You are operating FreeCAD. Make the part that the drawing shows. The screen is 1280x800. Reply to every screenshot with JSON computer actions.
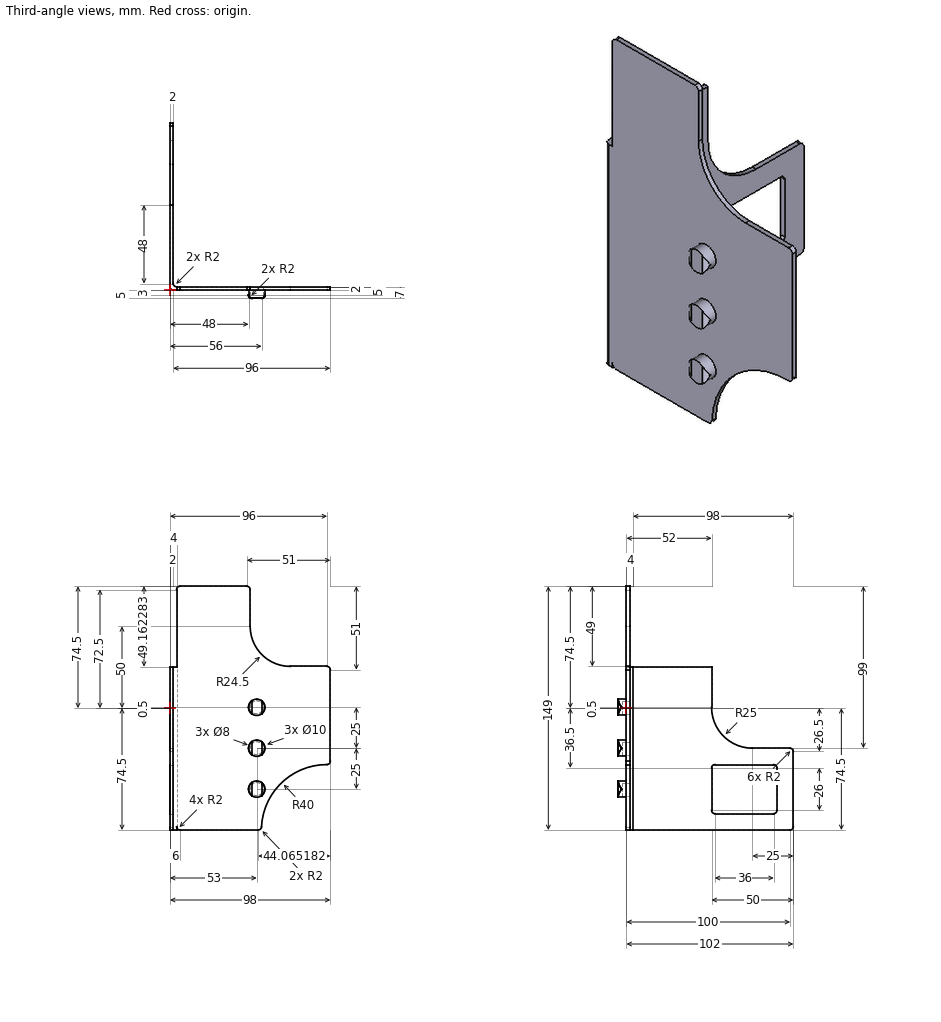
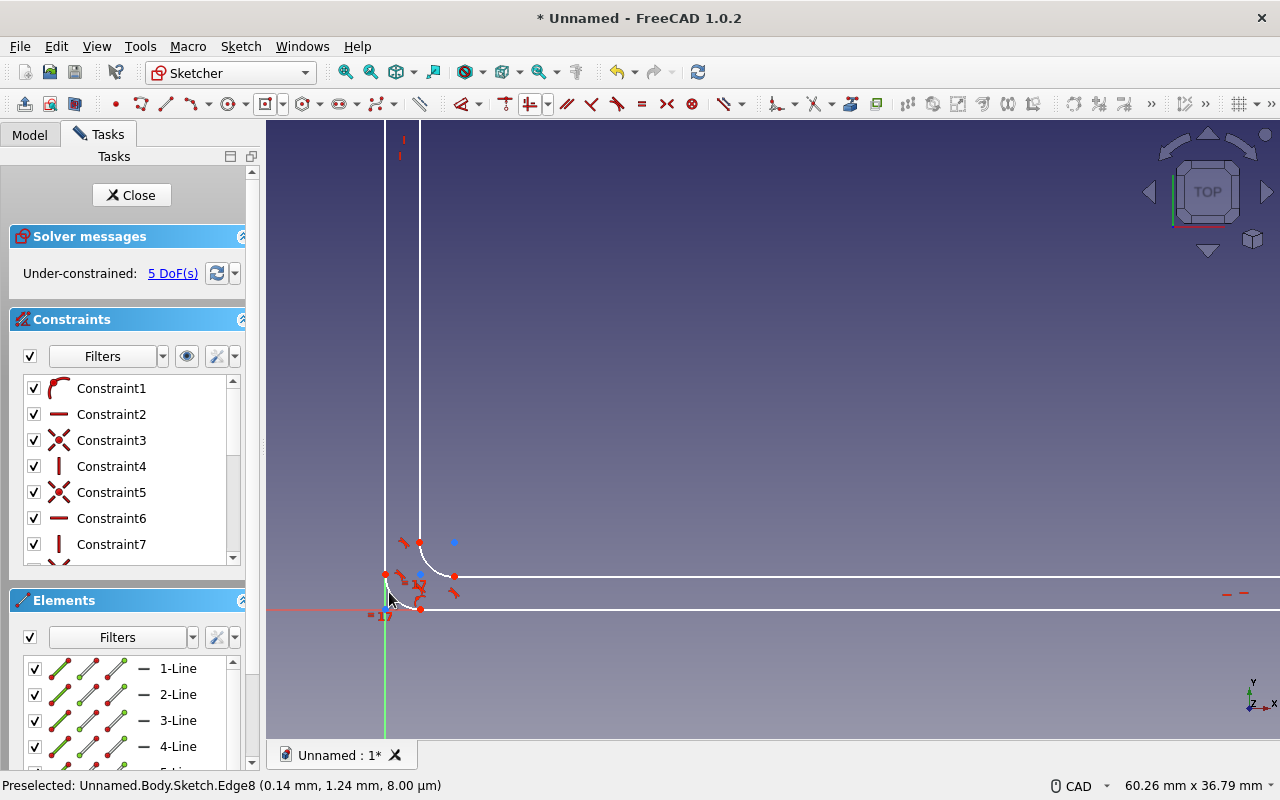
{"action": "left_click", "coordinate": [424, 558]}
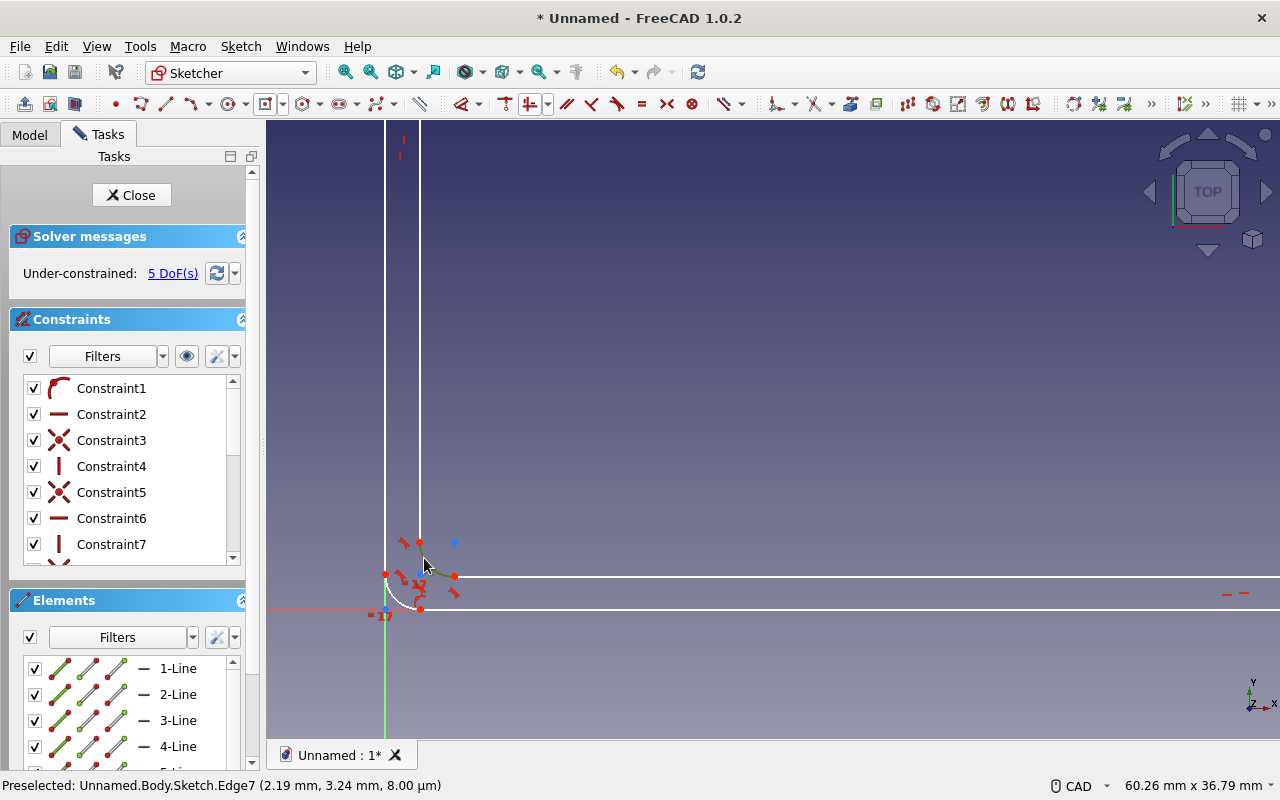
{"action": "key", "text": "k r"}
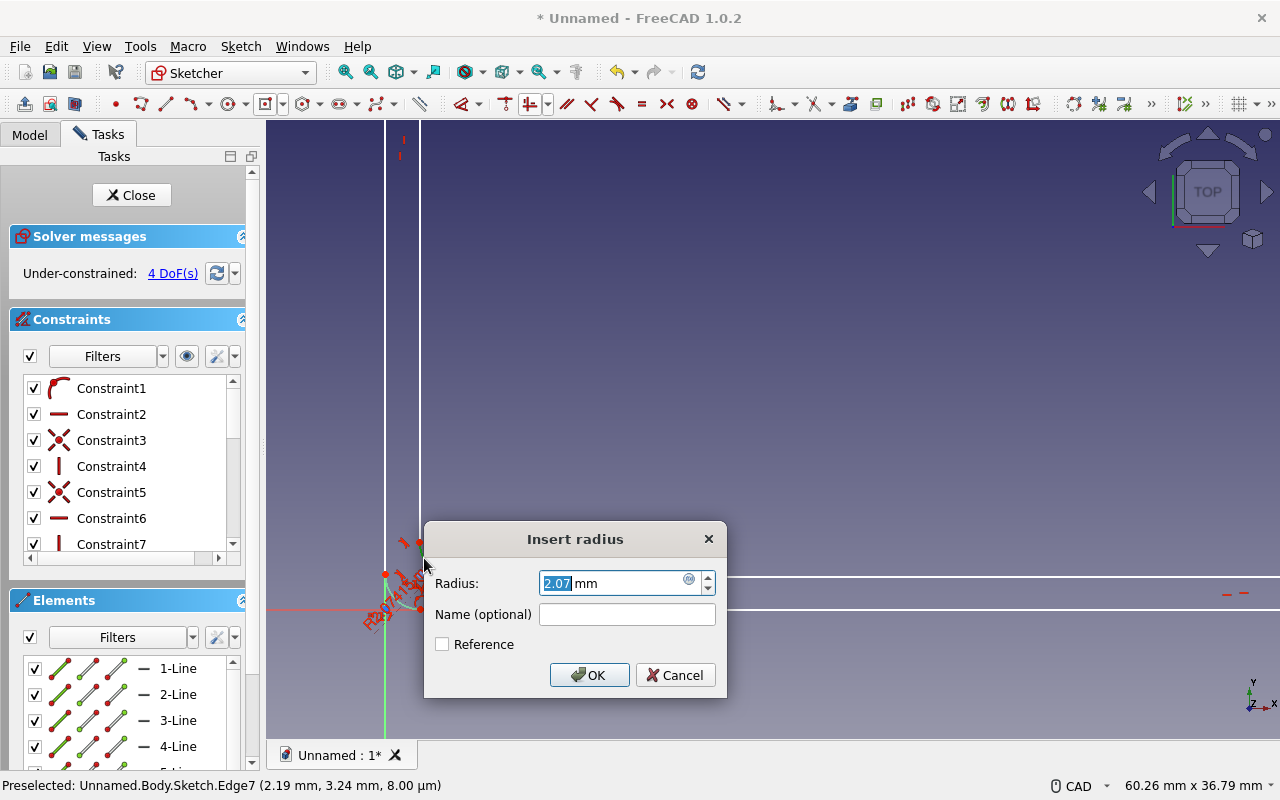
{"action": "type", "text": "2"}
{"action": "key", "text": "Return"}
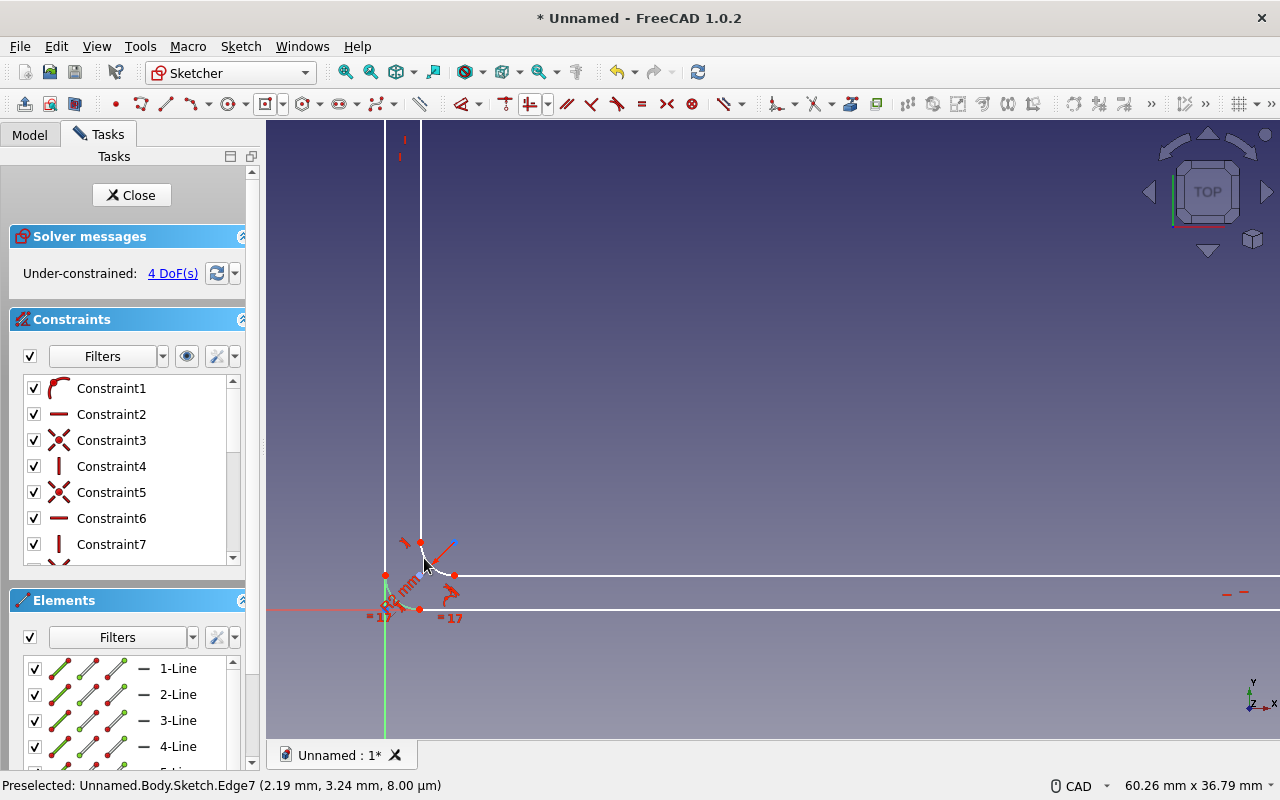
{"action": "scroll", "coordinate": [410, 579], "scroll_direction": "down", "scroll_amount": 5}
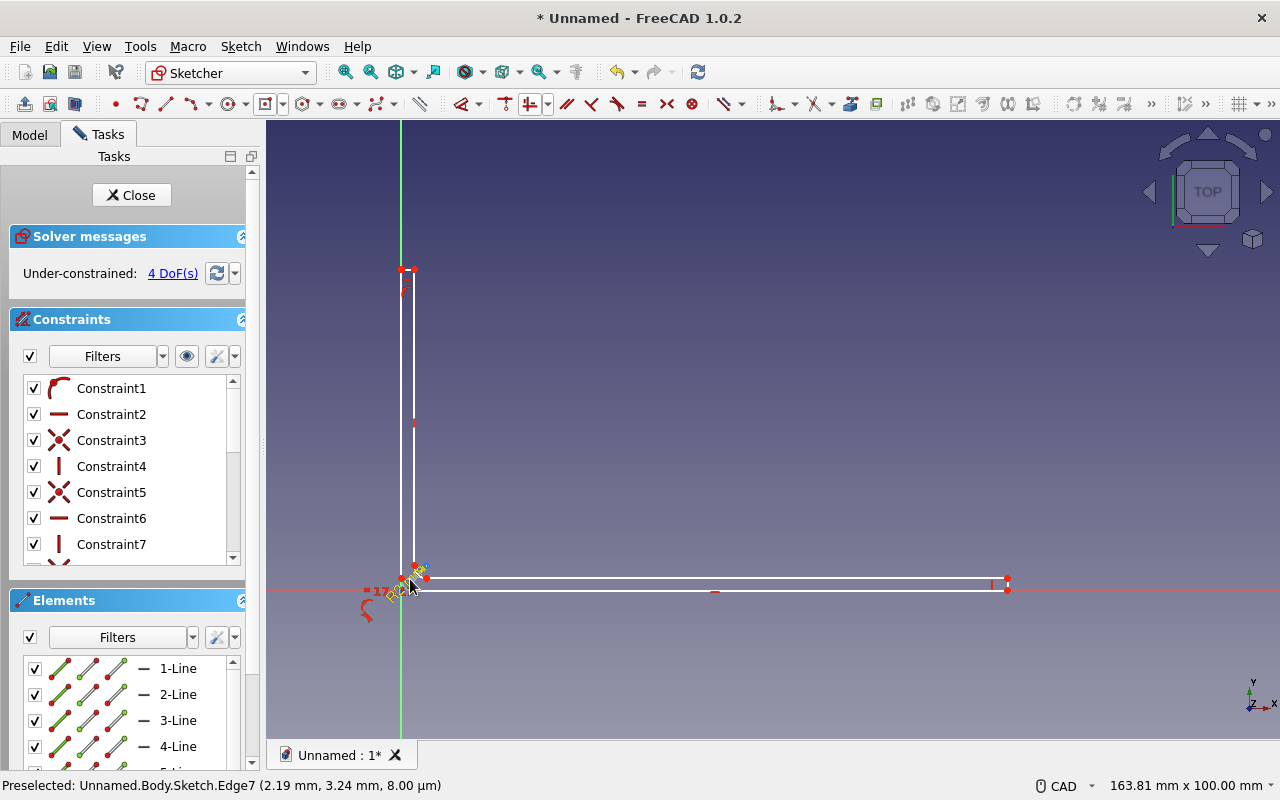
{"action": "scroll", "coordinate": [1008, 587], "scroll_direction": "up", "scroll_amount": 7}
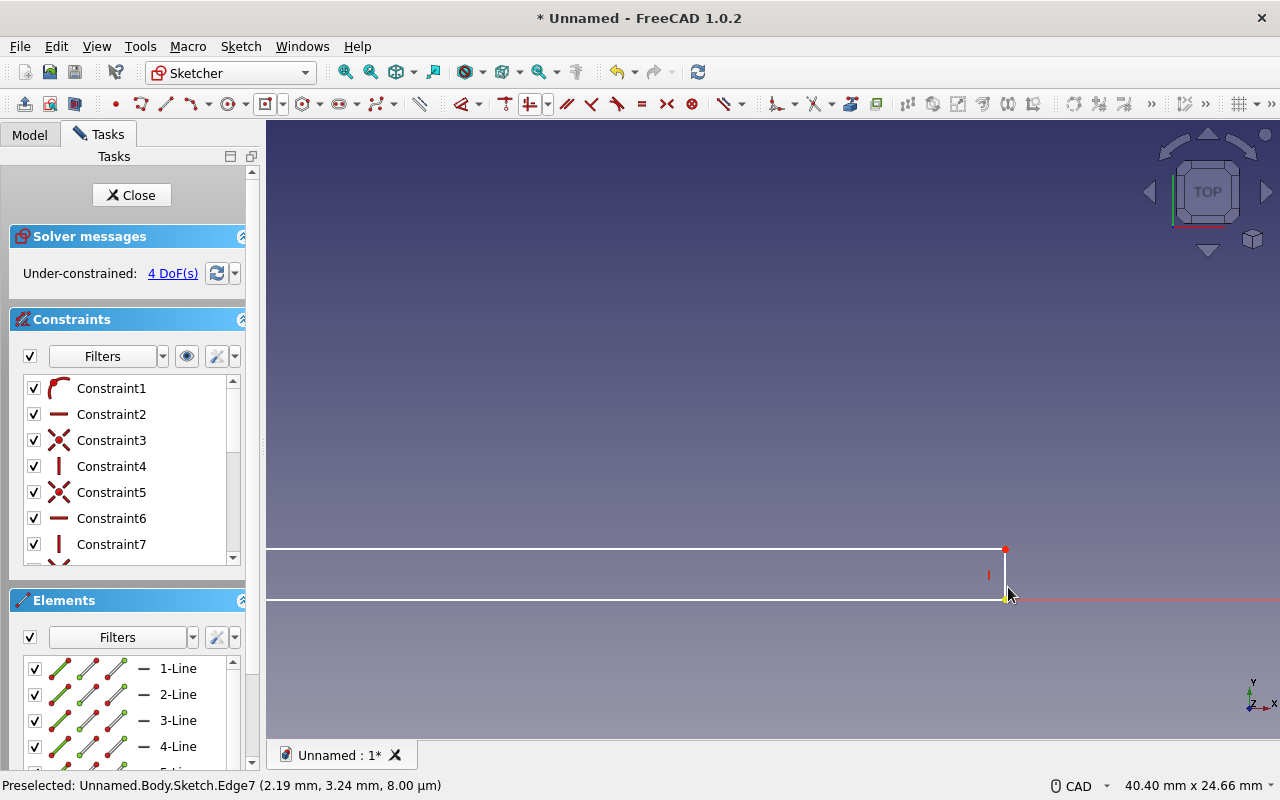
{"action": "left_click", "coordinate": [1005, 585]}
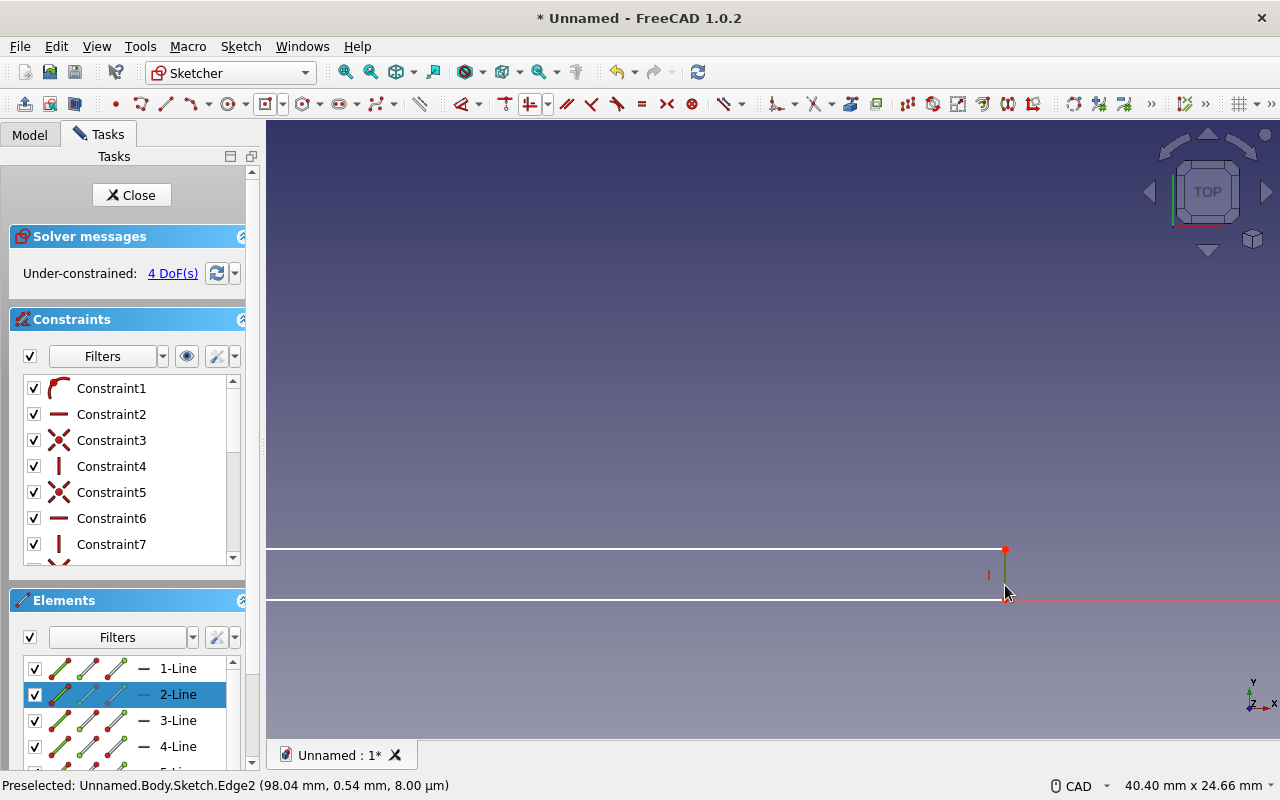
{"action": "key", "text": "i"}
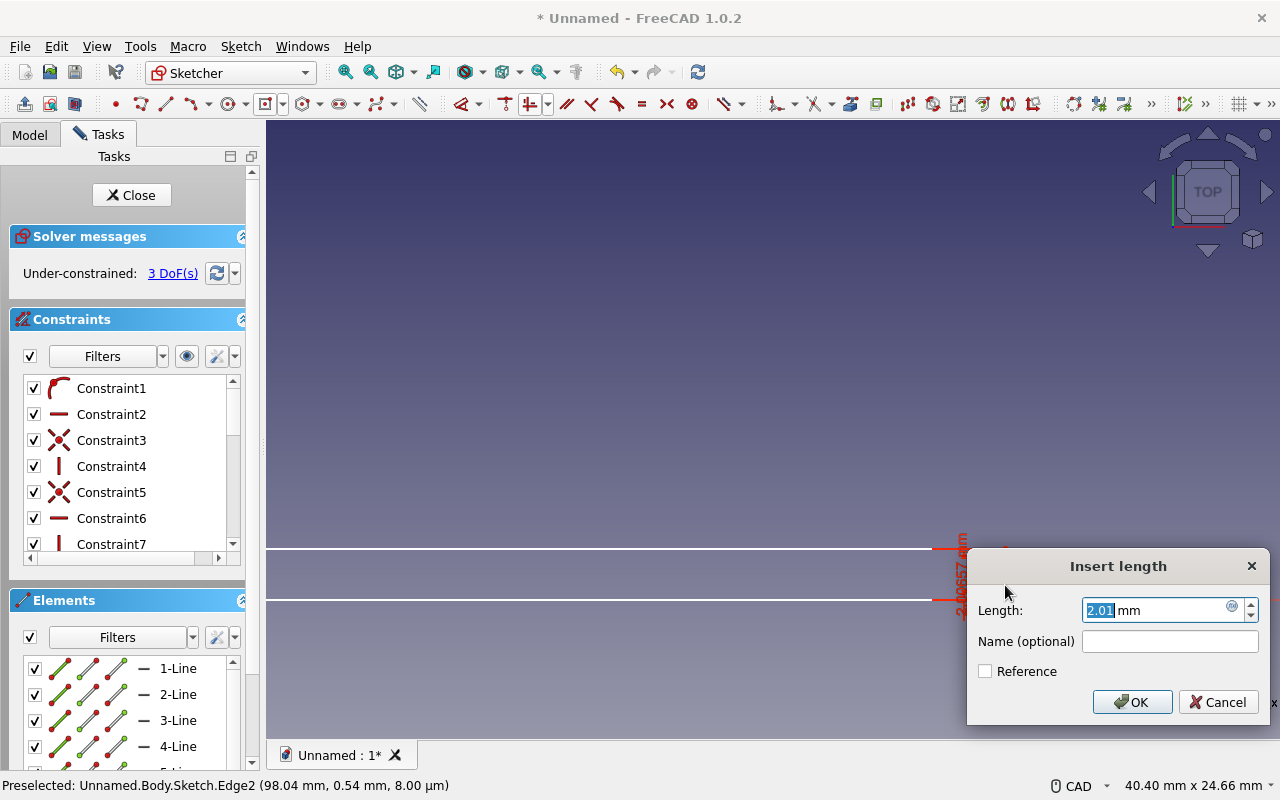
{"action": "type", "text": "2"}
{"action": "key", "text": "Return"}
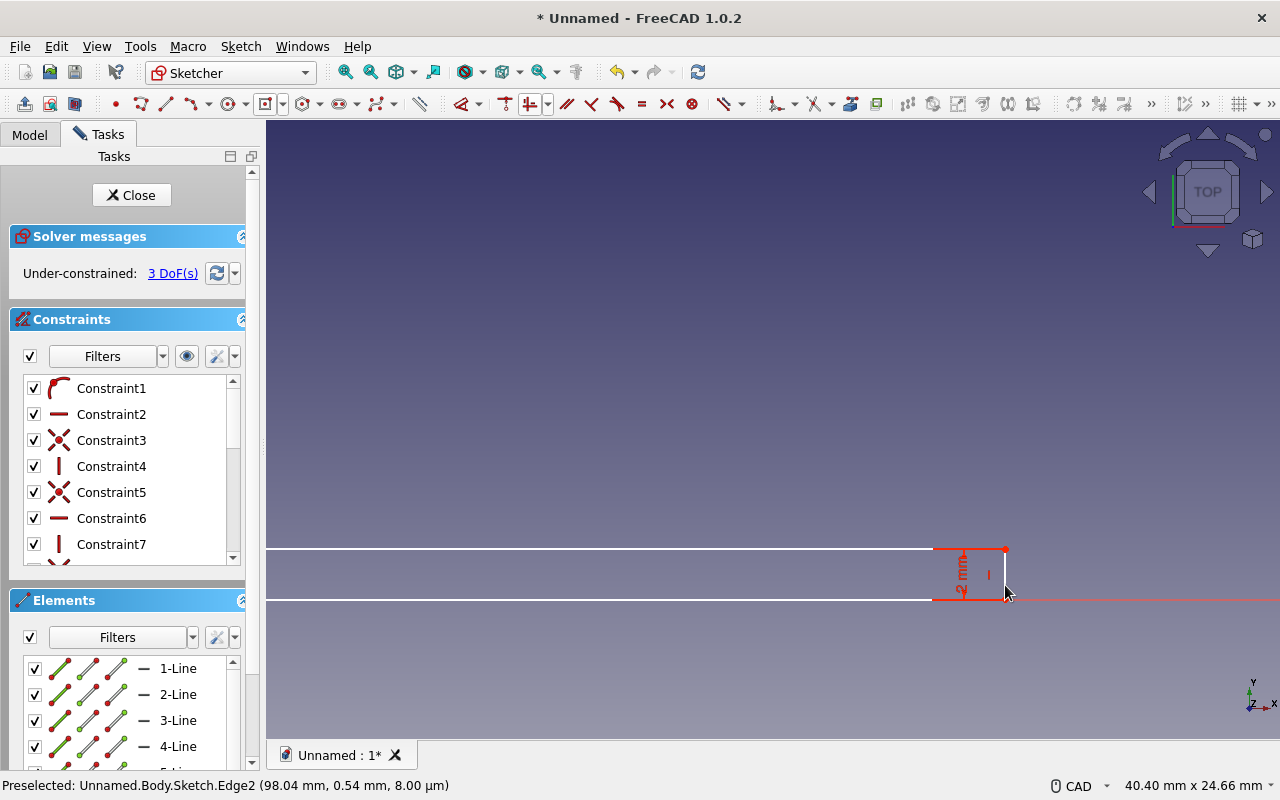
{"action": "scroll", "coordinate": [1009, 587], "scroll_direction": "down", "scroll_amount": 7}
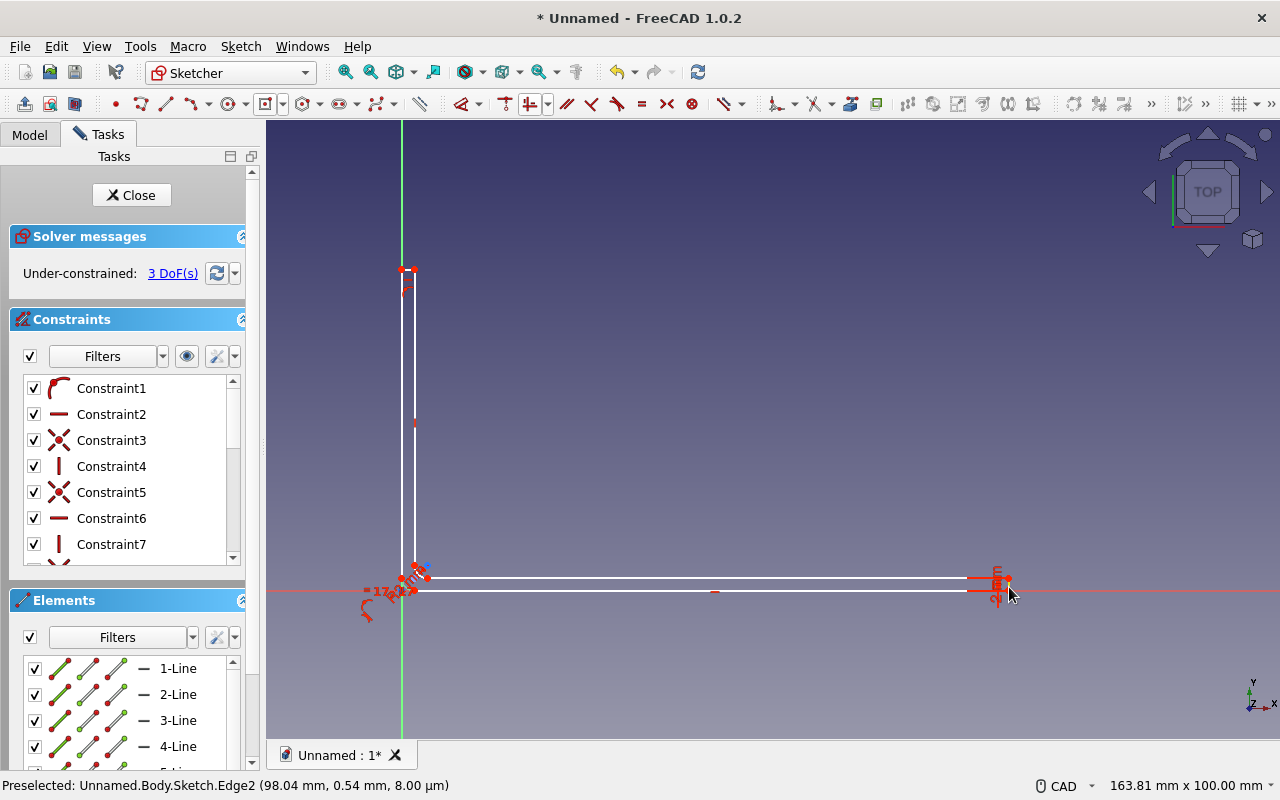
{"action": "scroll", "coordinate": [411, 270], "scroll_direction": "up", "scroll_amount": 7}